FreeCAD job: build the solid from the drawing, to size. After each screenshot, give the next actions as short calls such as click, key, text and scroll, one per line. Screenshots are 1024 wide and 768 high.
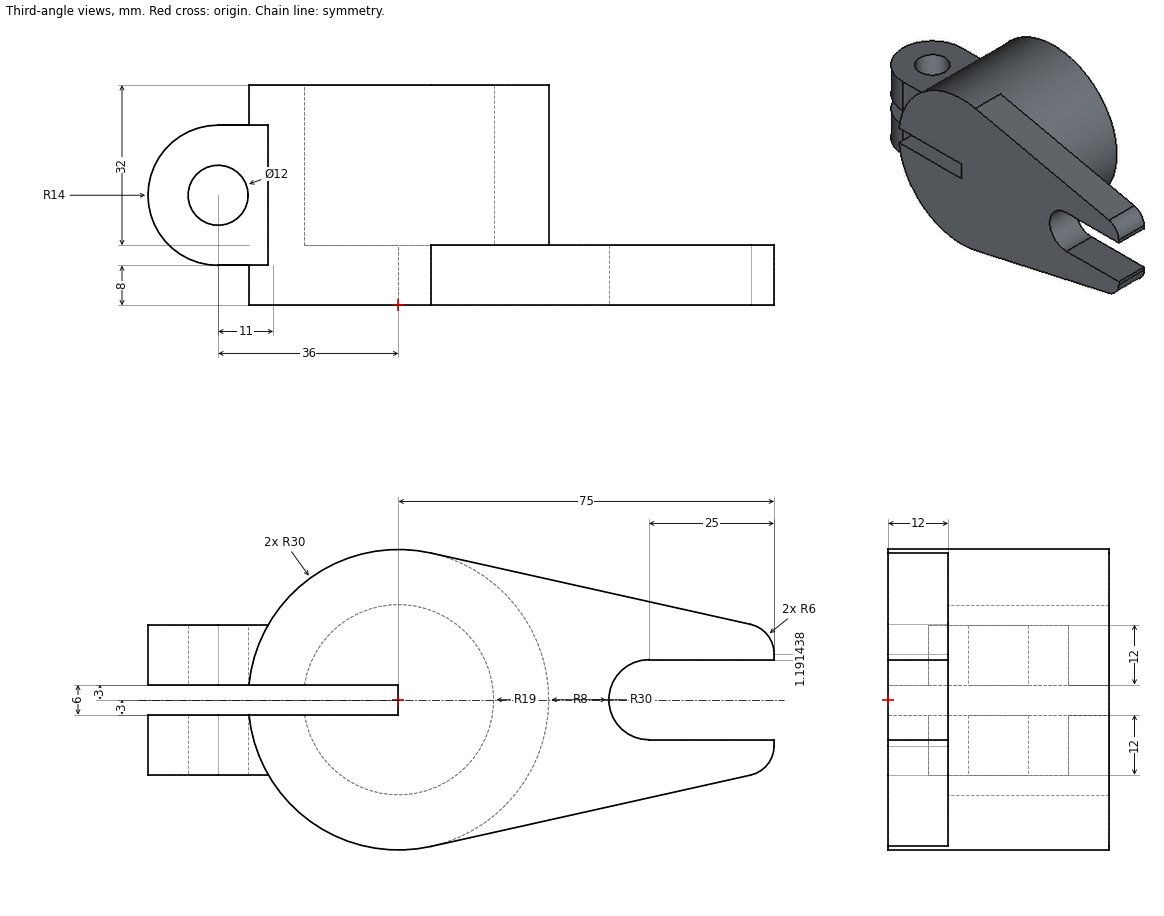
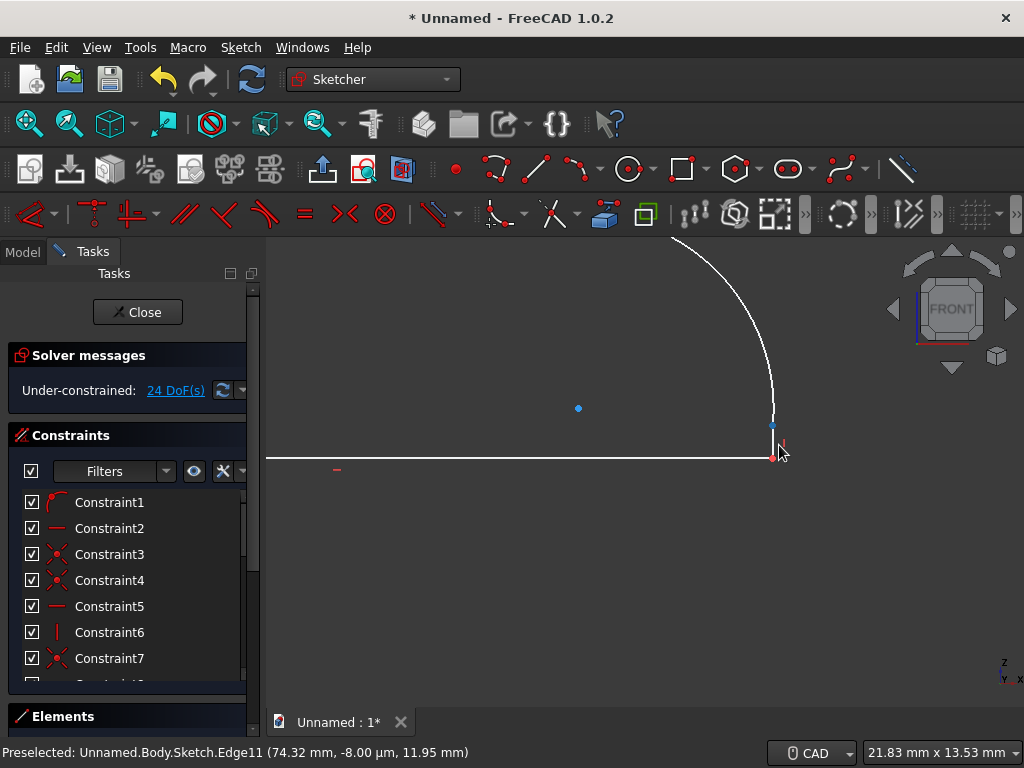
click(773, 442)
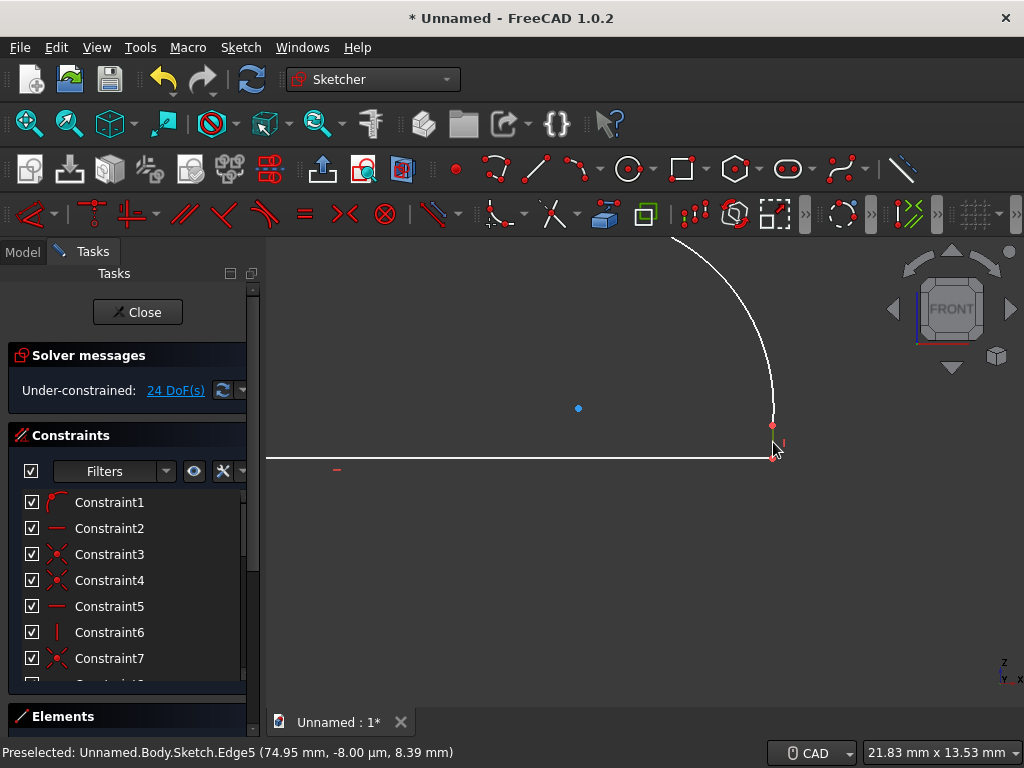
scroll(779, 439, down, 11)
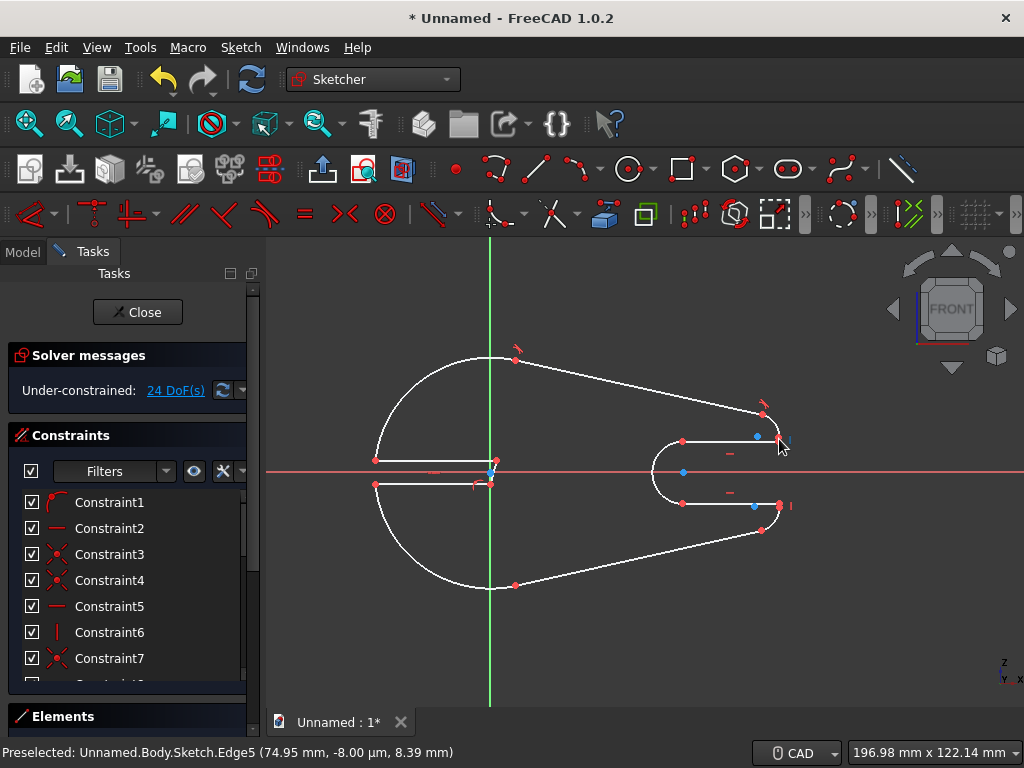
scroll(778, 429, up, 2)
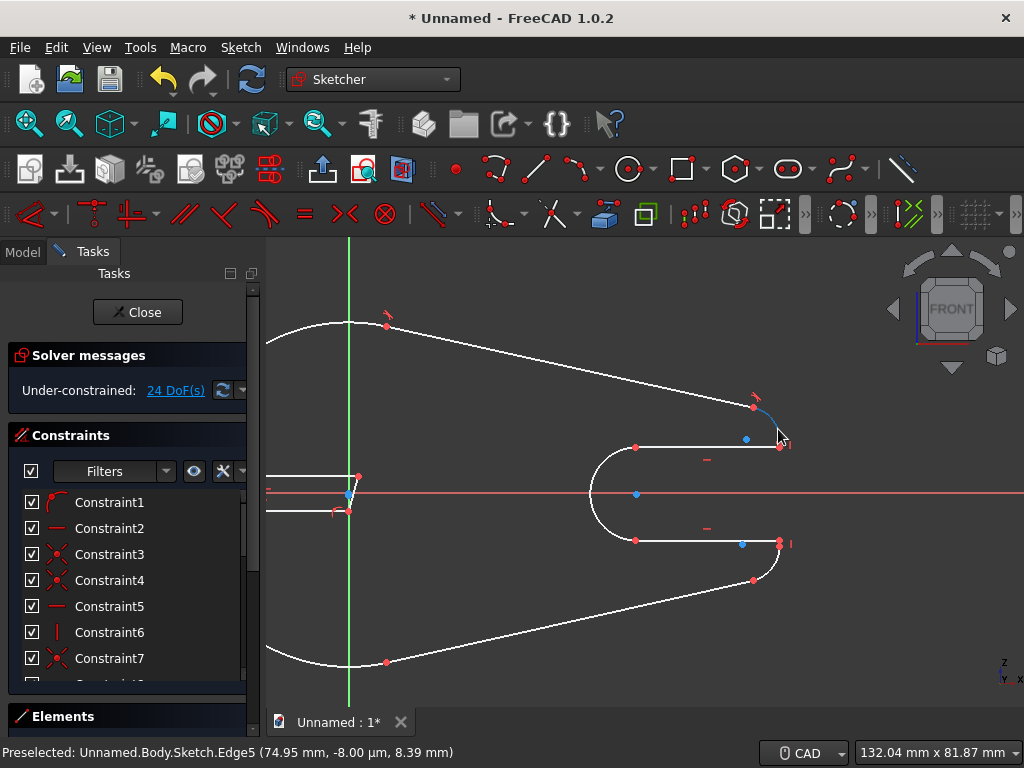
click(777, 428)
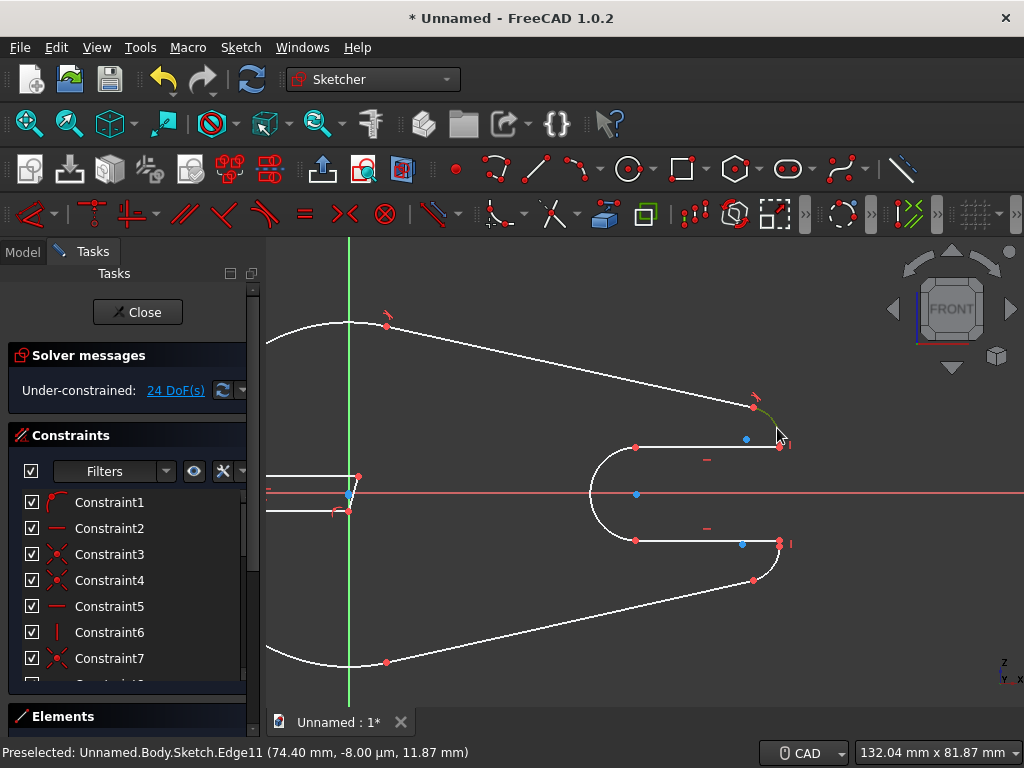
key(t)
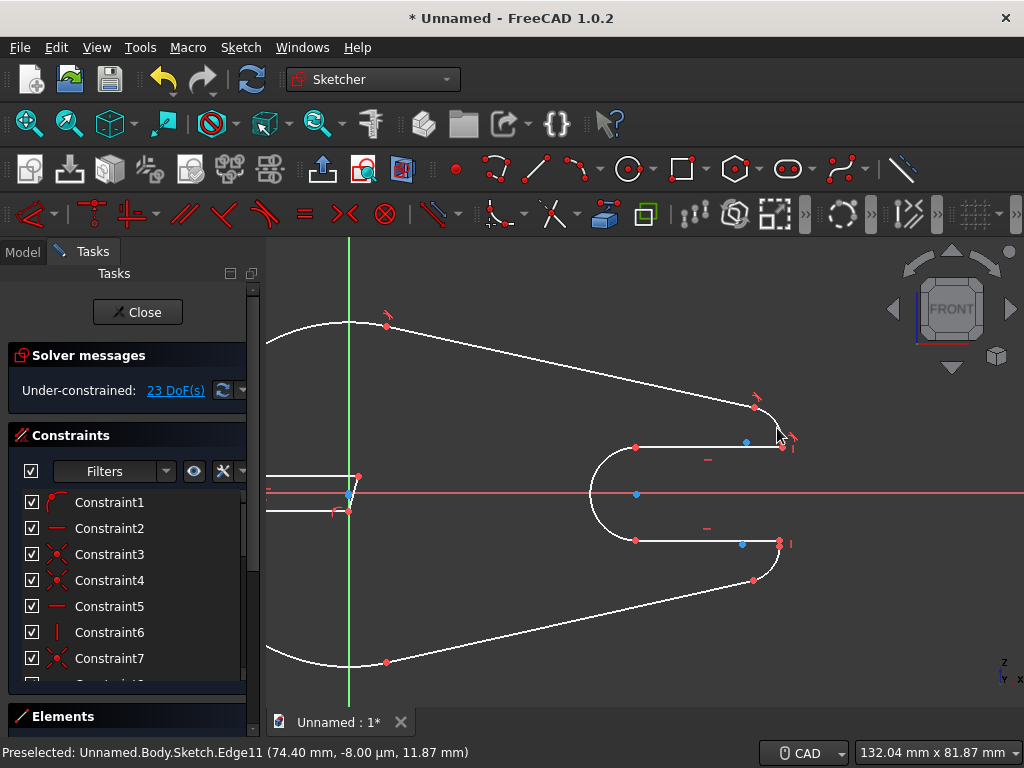
click(738, 447)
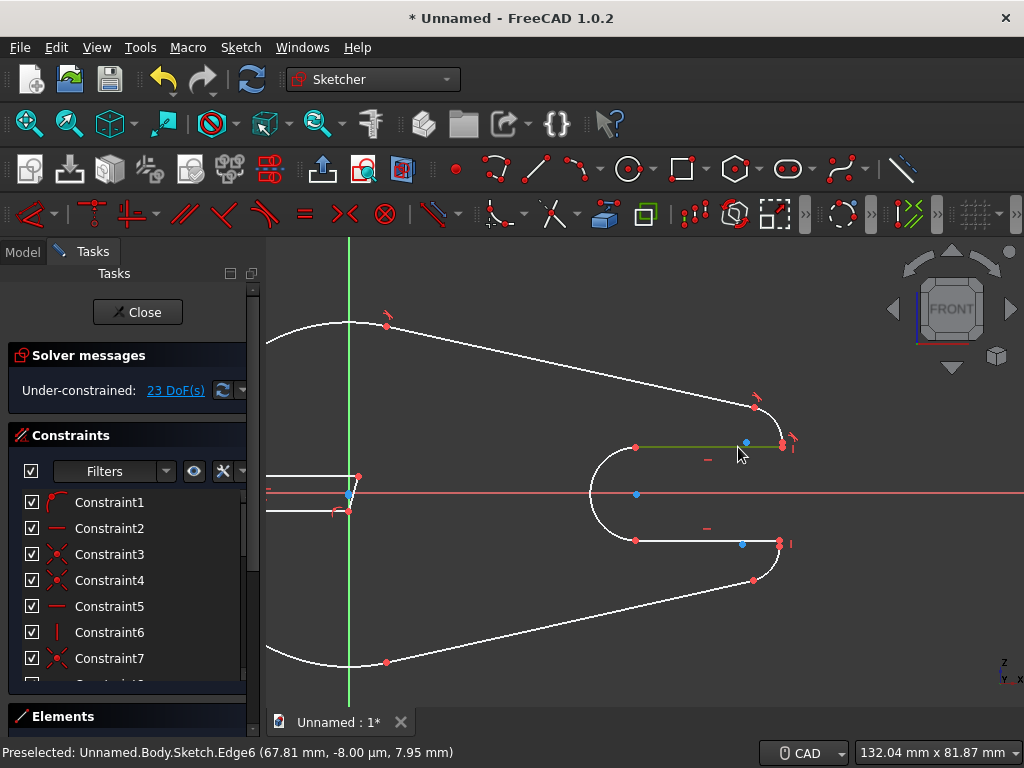
click(599, 467)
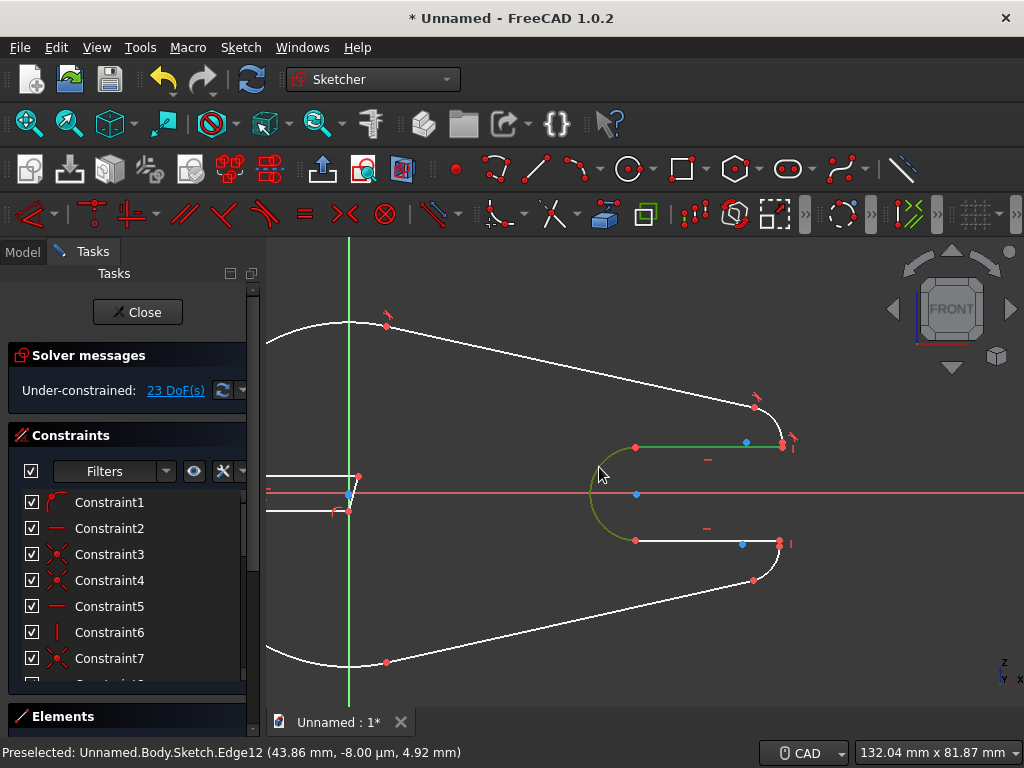
click(266, 214)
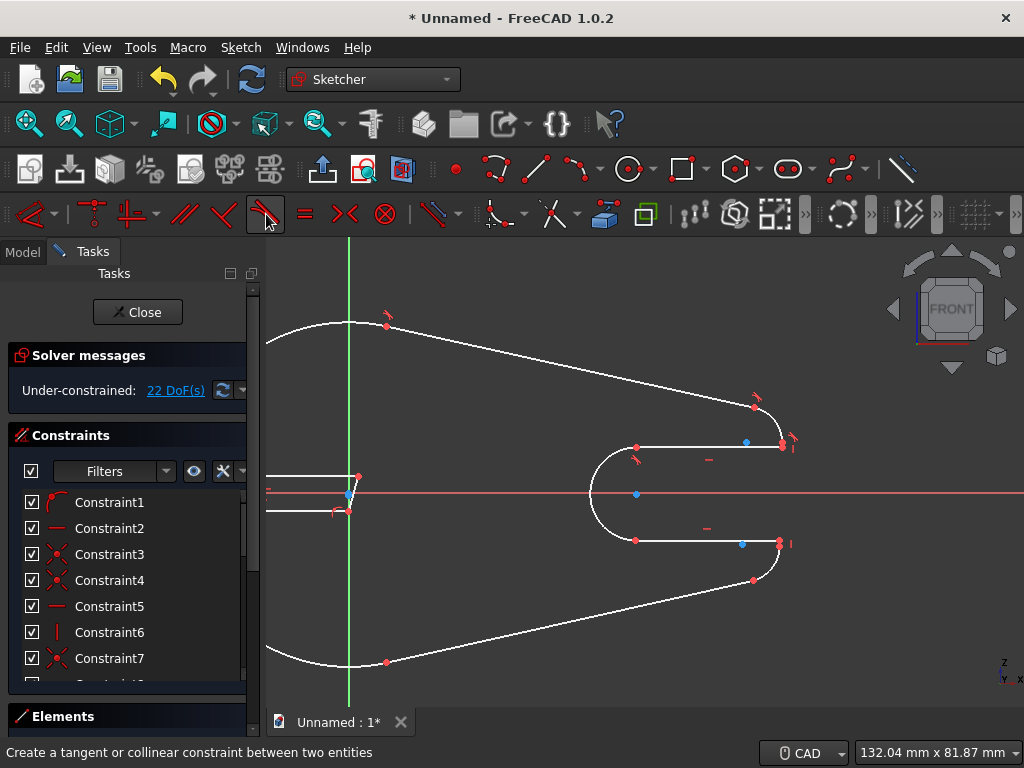
click(679, 541)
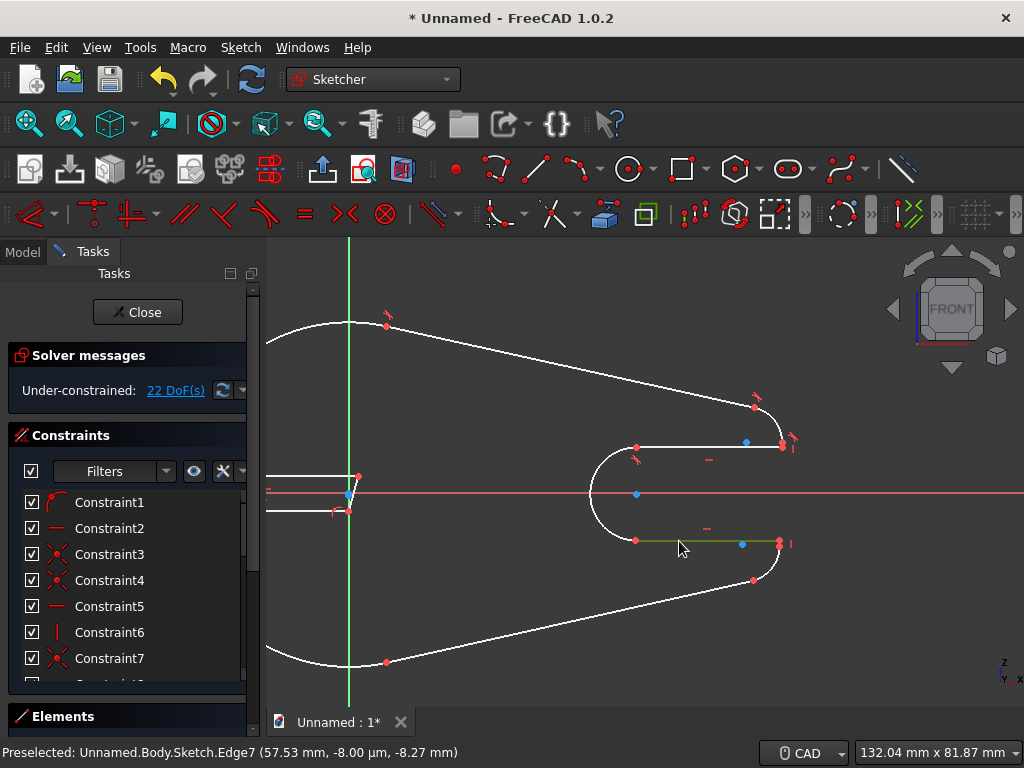
click(600, 466)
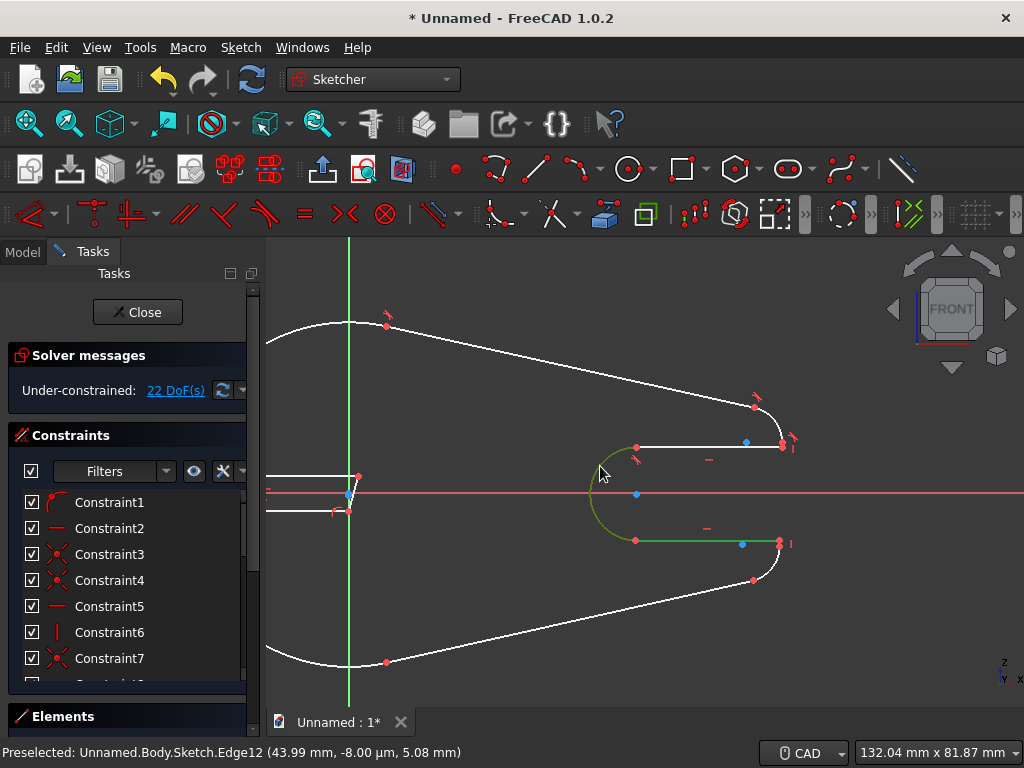
key(t)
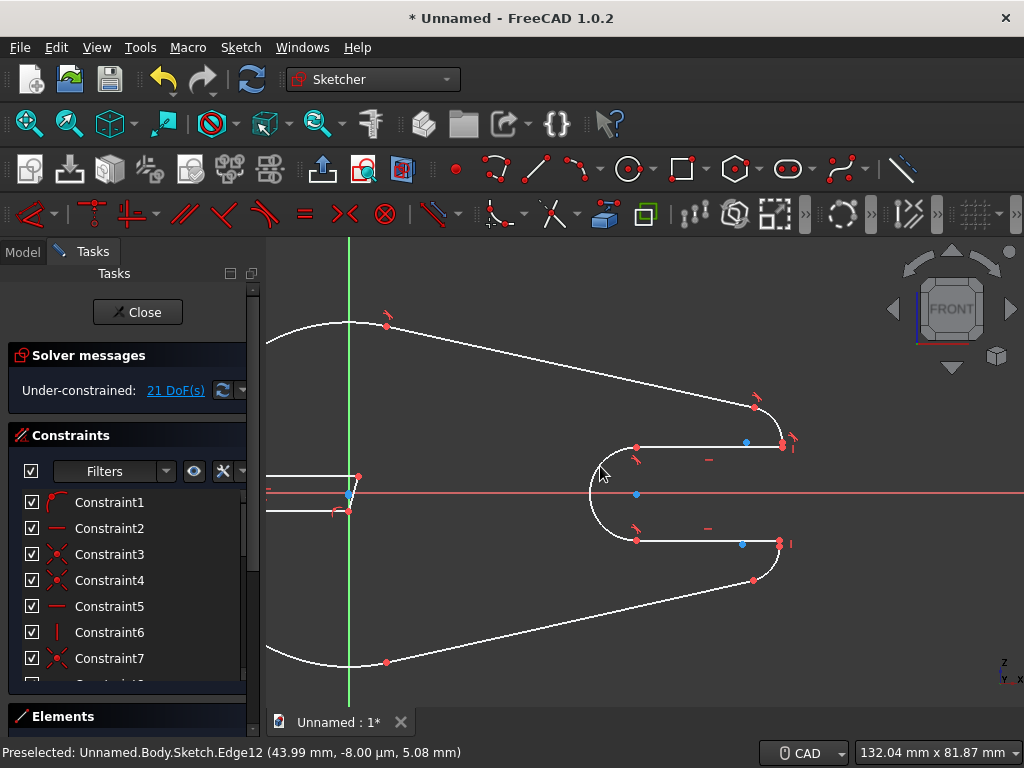
scroll(780, 543, up, 9)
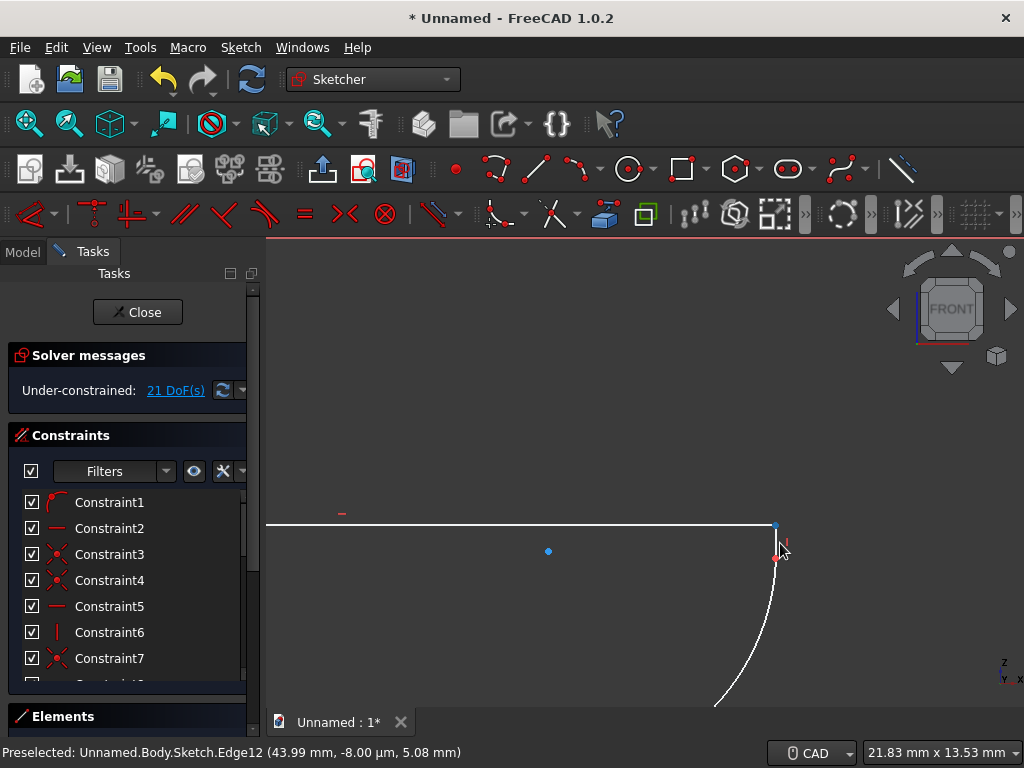
click(776, 542)